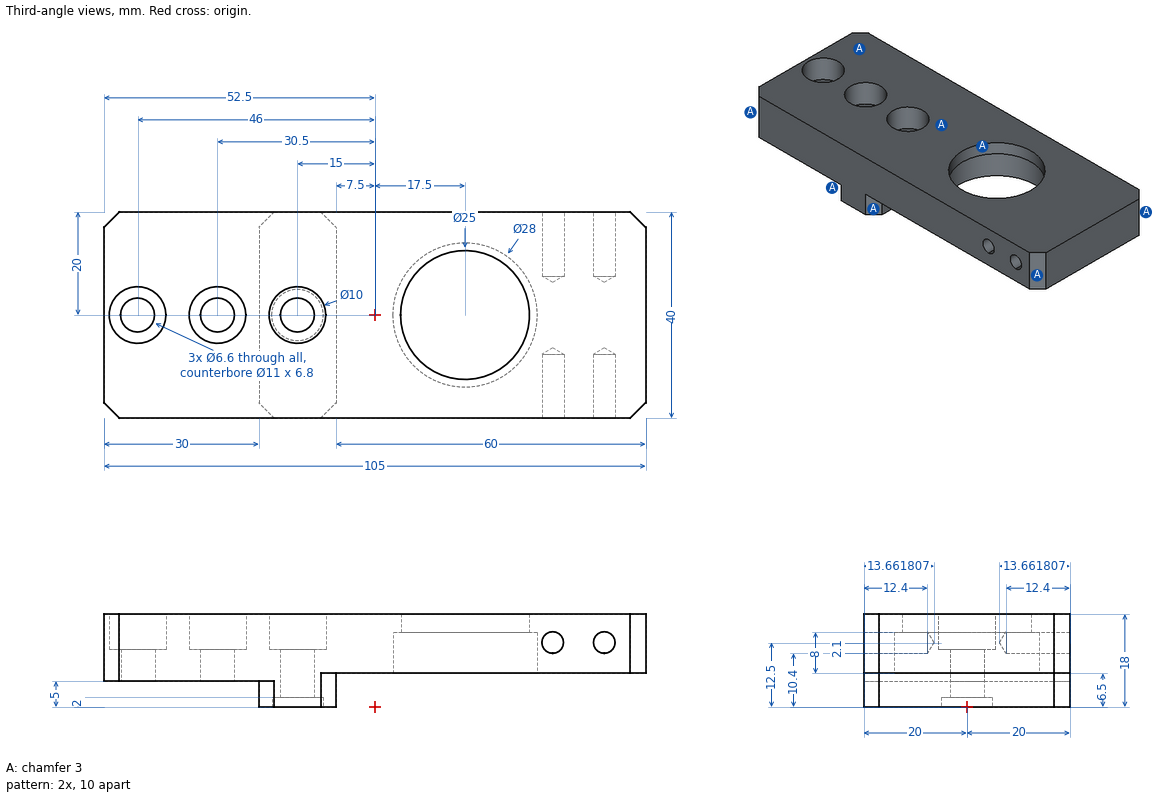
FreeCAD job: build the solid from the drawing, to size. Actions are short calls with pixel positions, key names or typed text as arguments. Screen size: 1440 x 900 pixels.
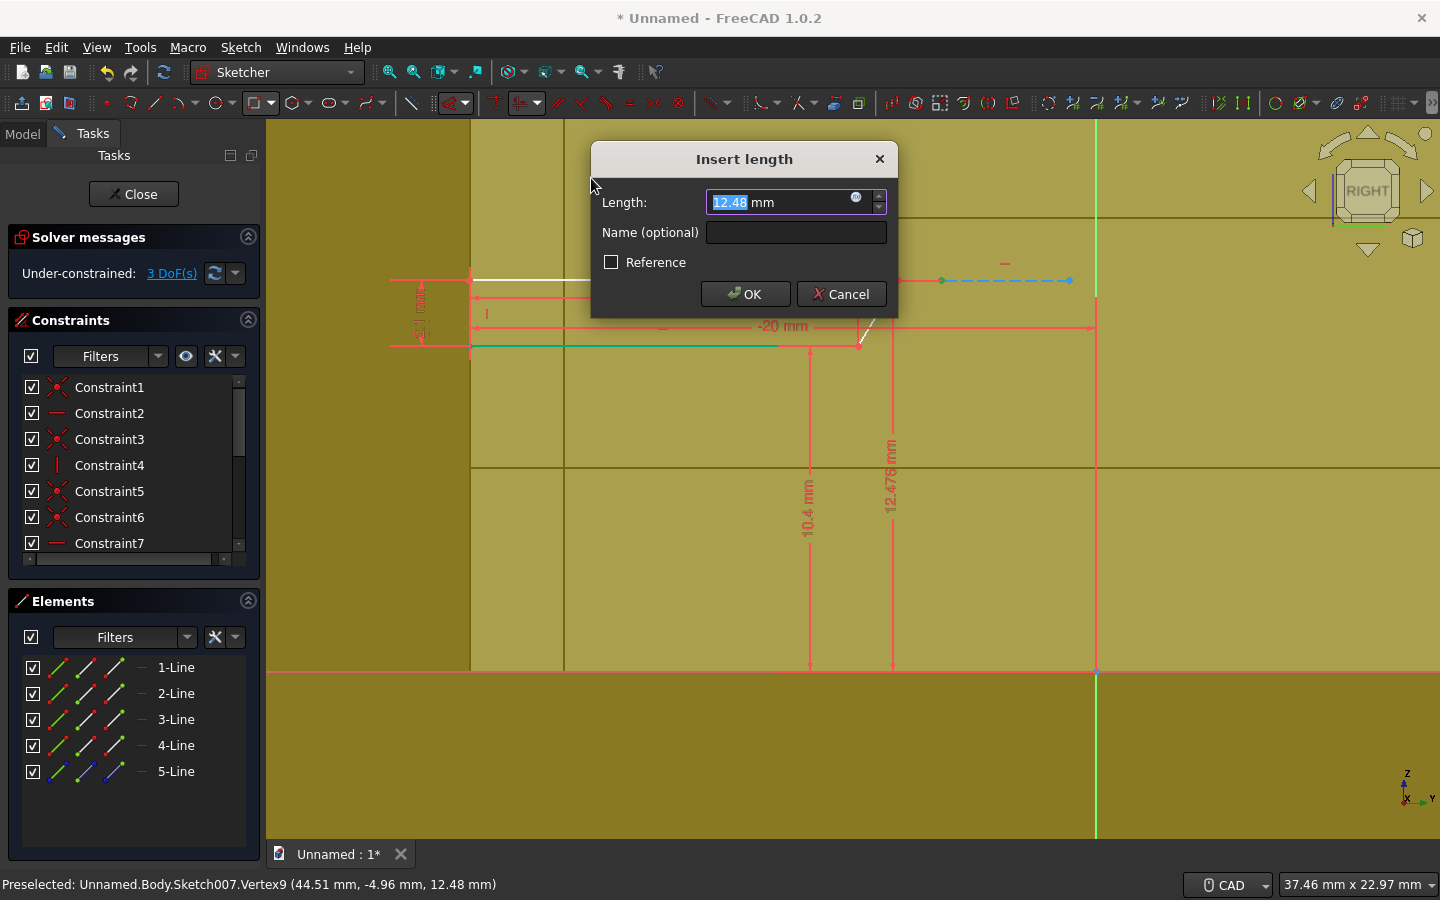
text(12.5)
key(Return)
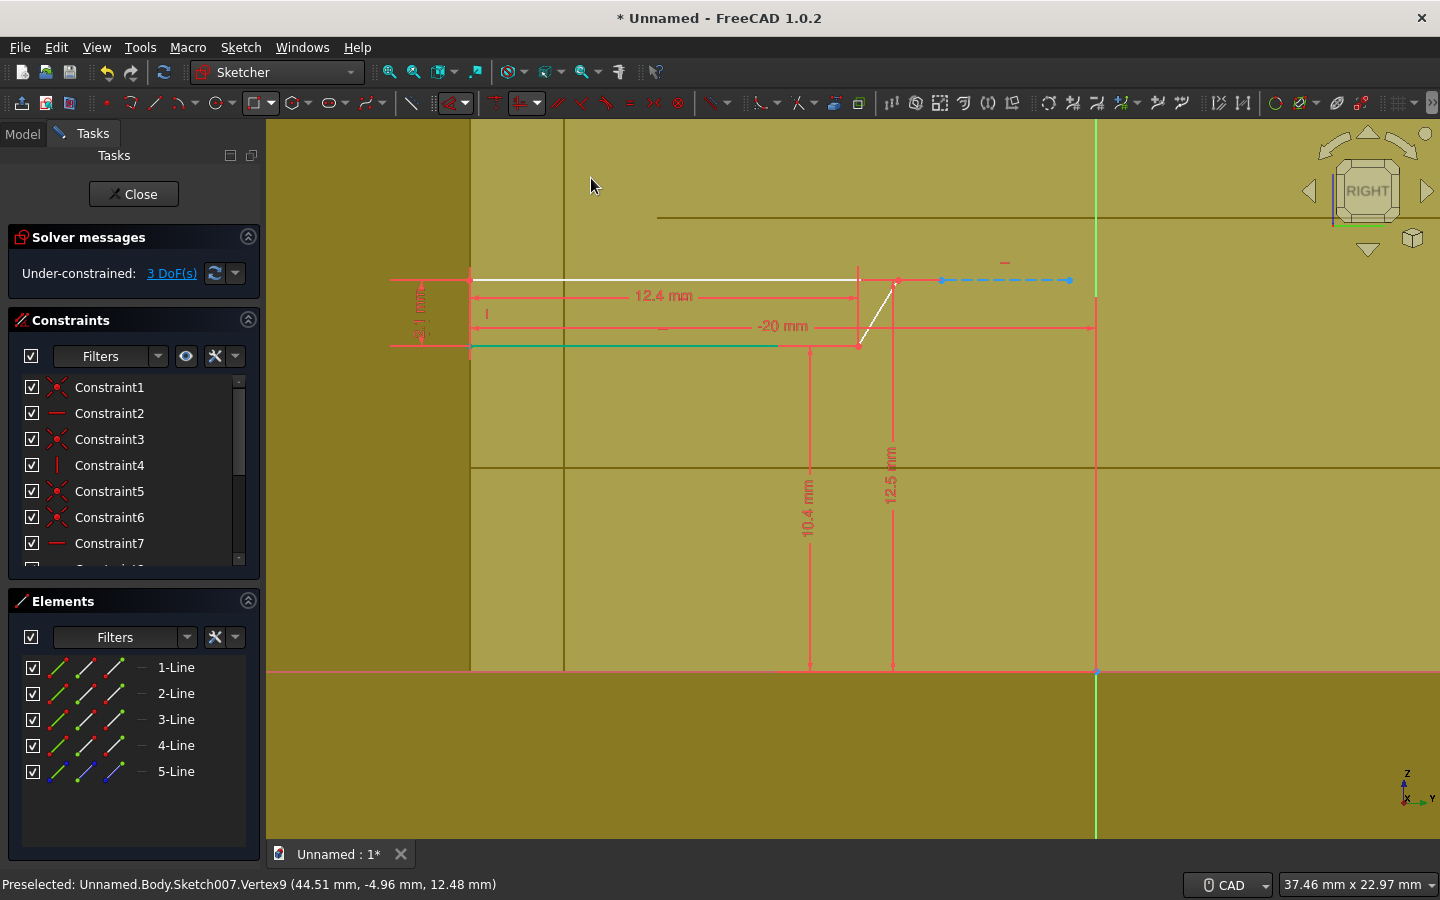
click(769, 280)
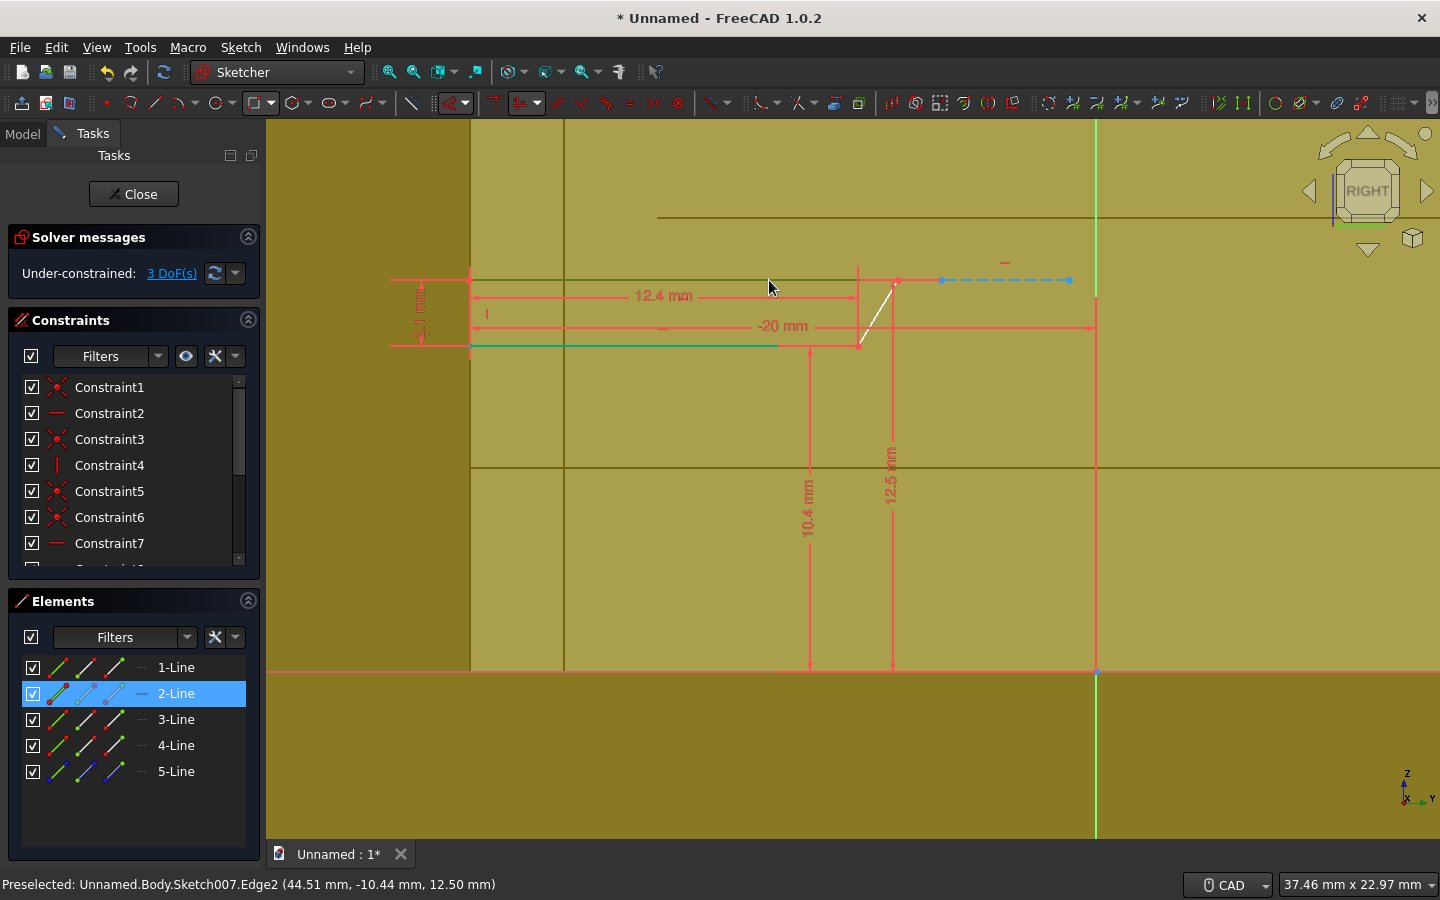
click(468, 104)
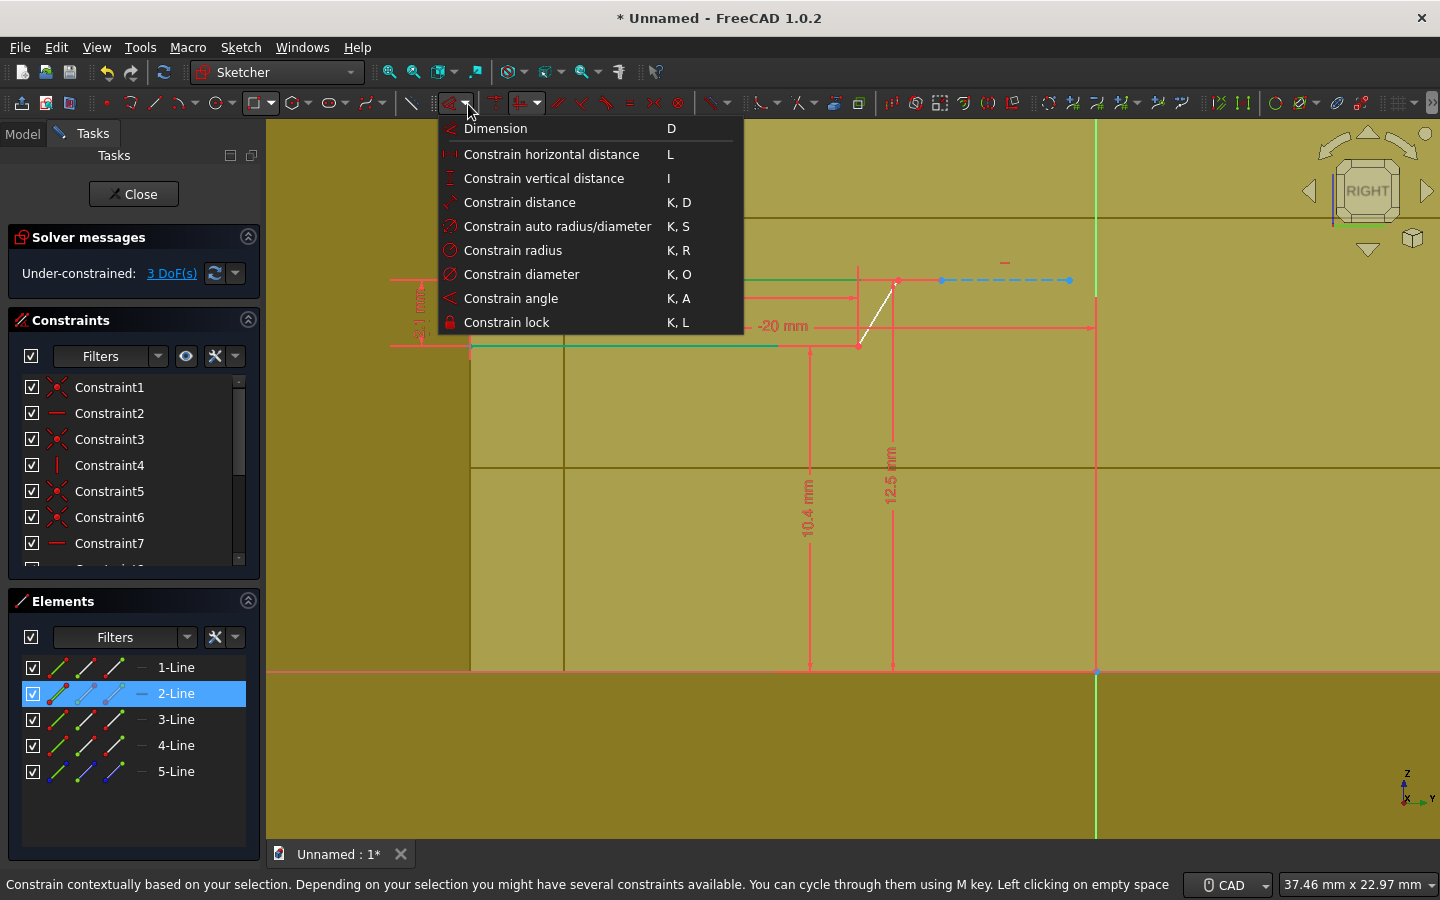
click(591, 154)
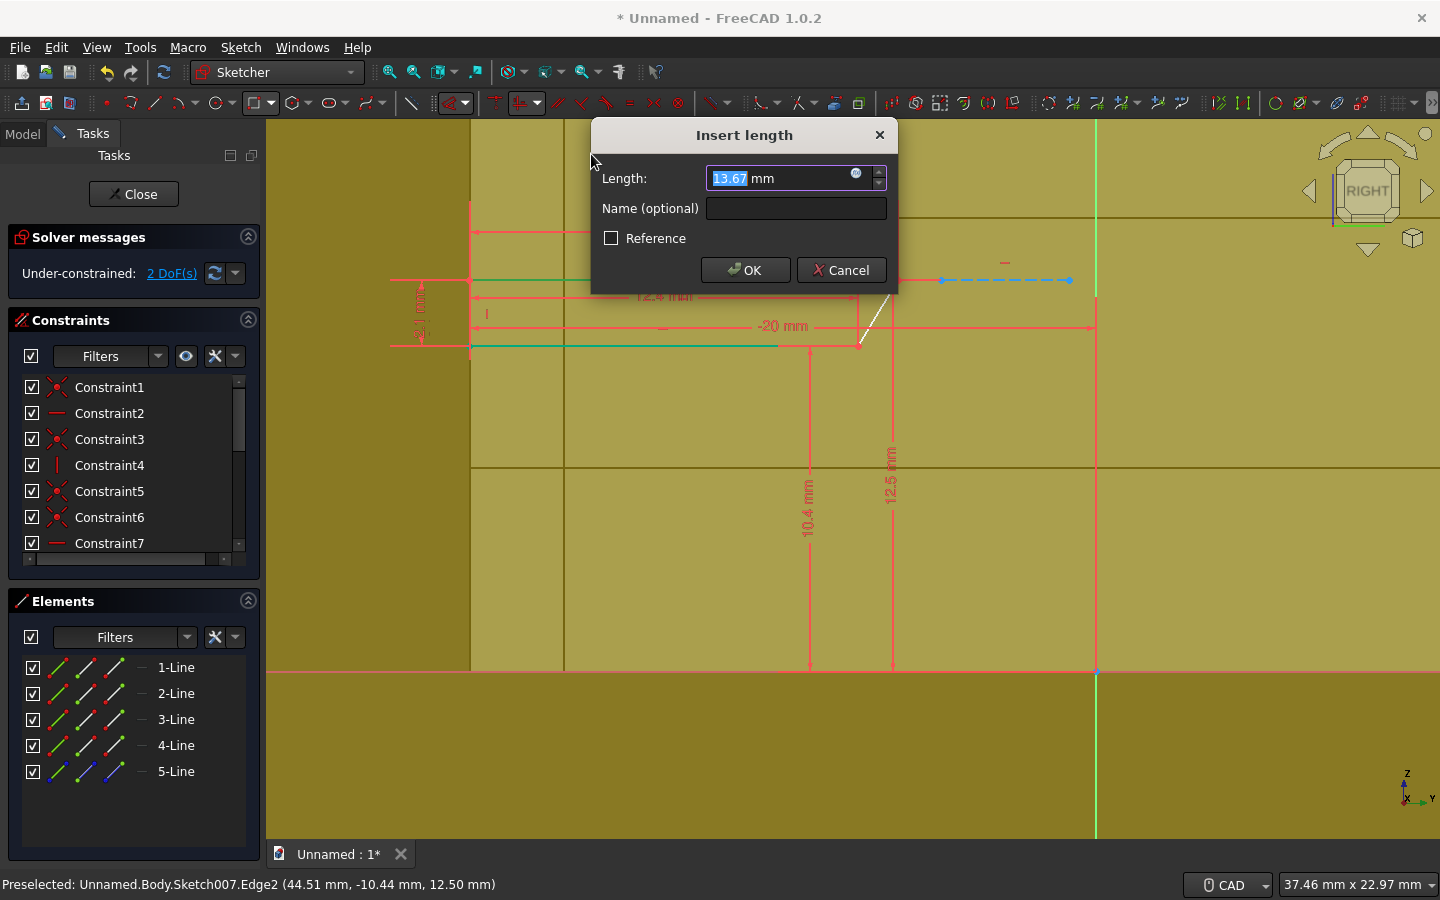
text(13.661807)
key(Return)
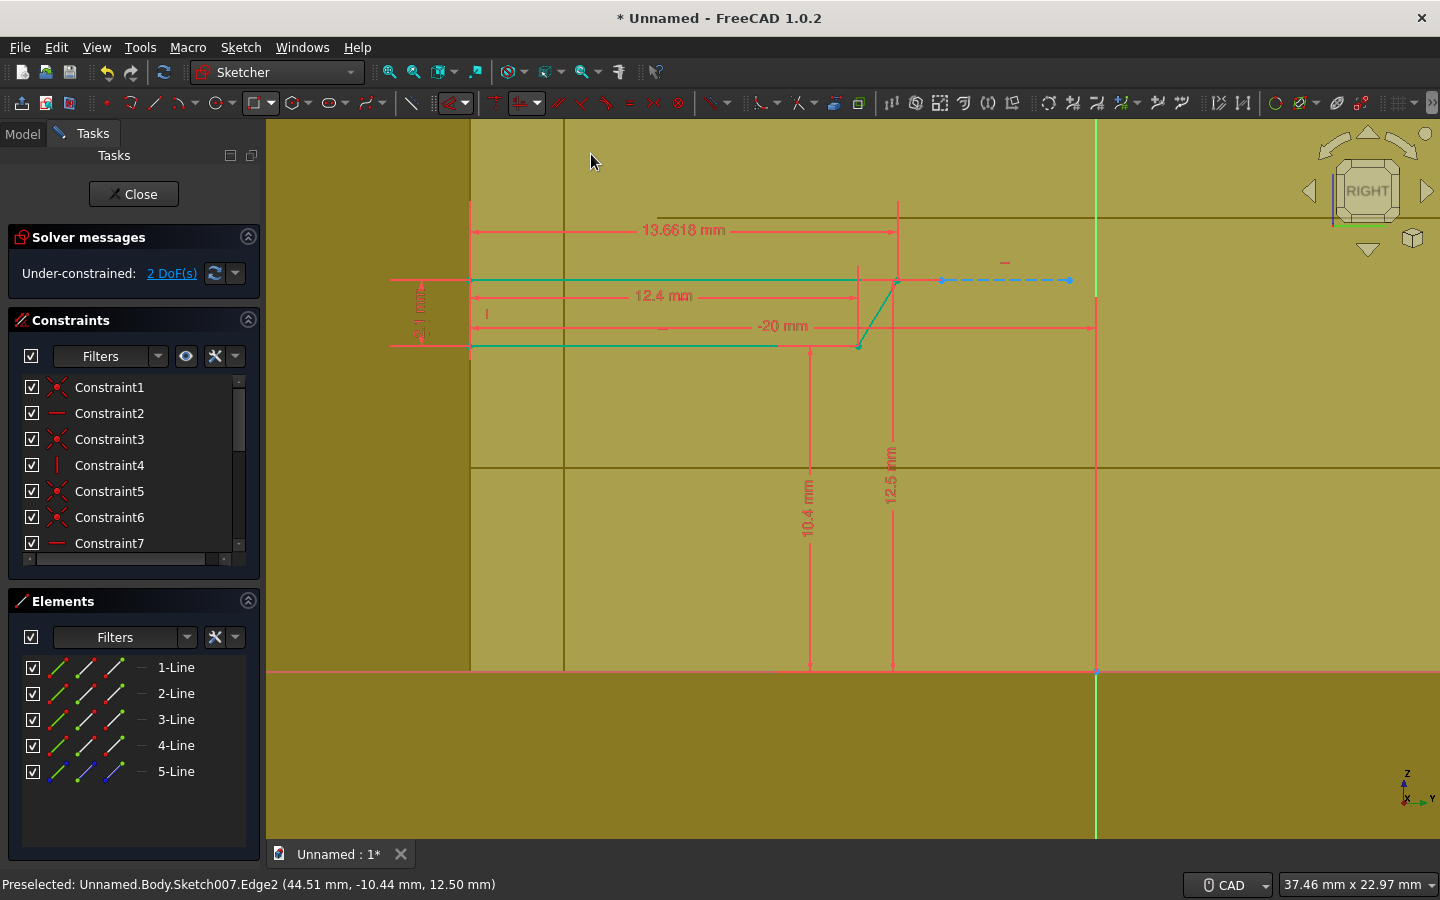
click(134, 194)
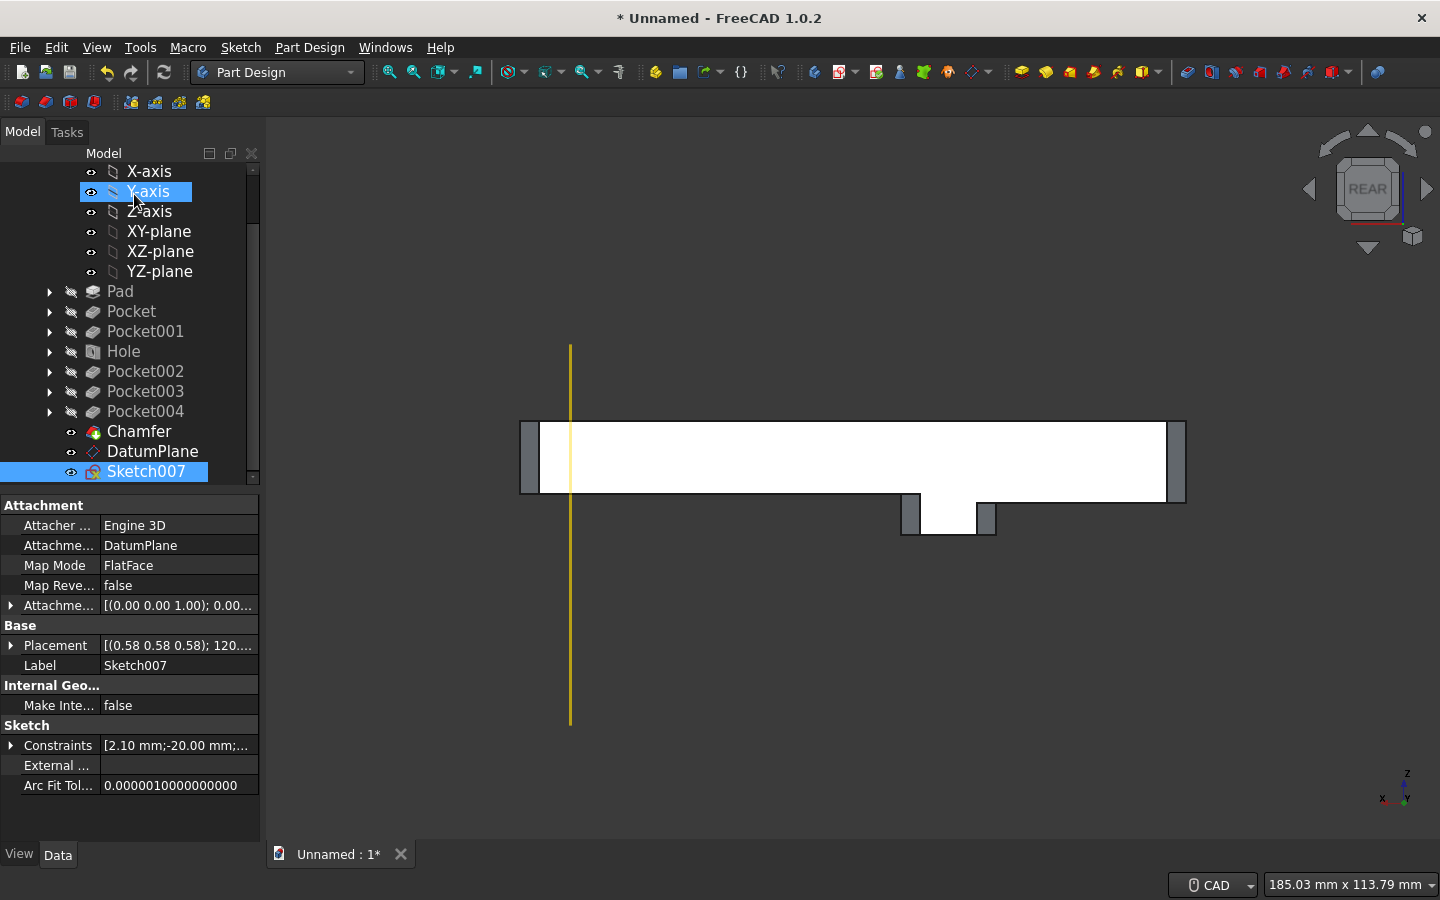
click(1236, 72)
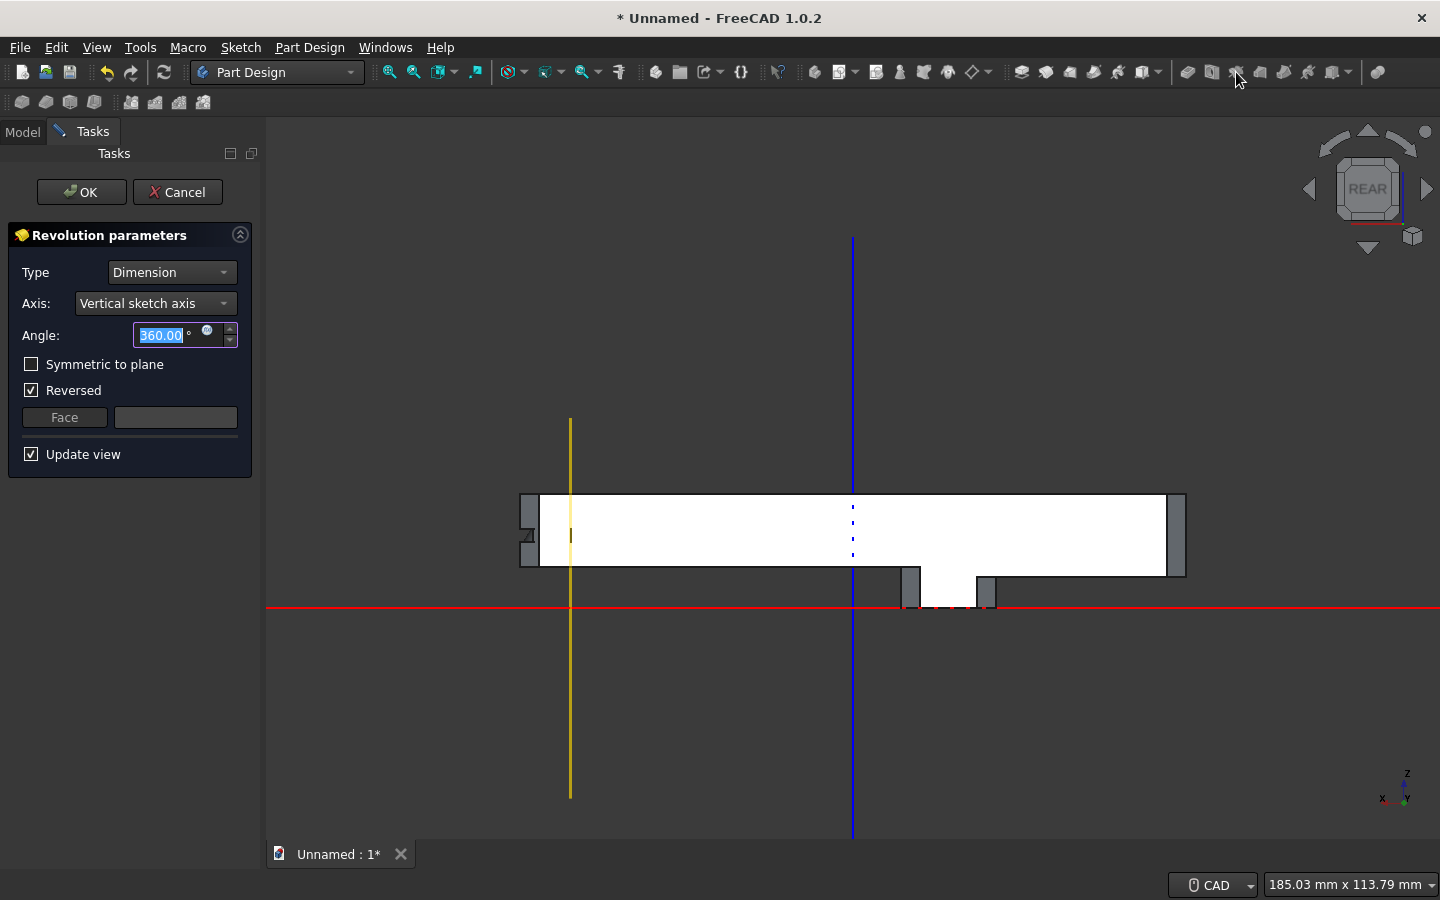
click(156, 304)